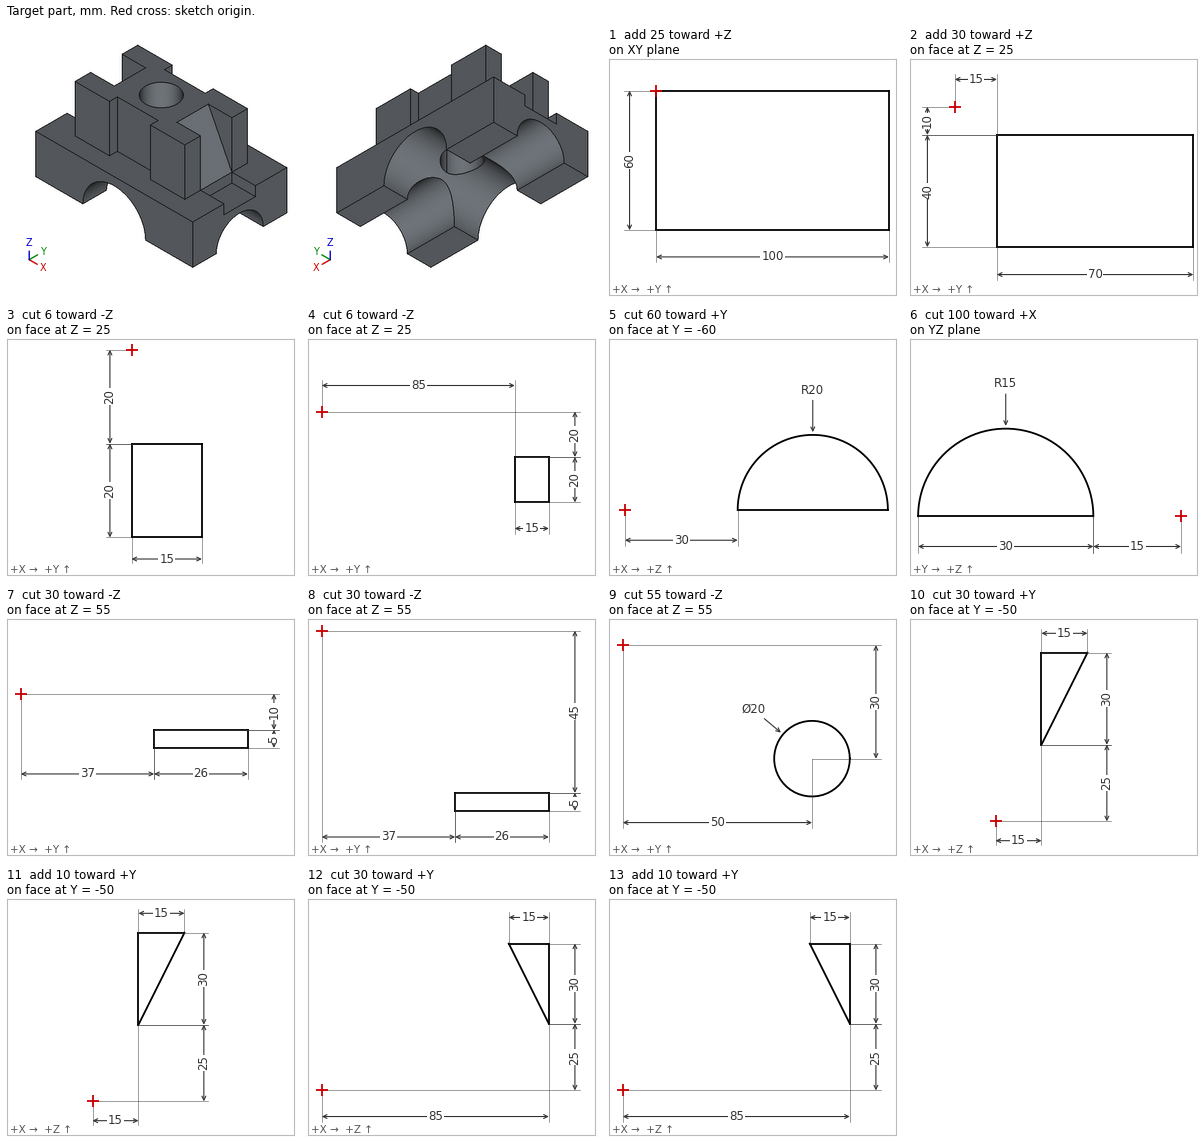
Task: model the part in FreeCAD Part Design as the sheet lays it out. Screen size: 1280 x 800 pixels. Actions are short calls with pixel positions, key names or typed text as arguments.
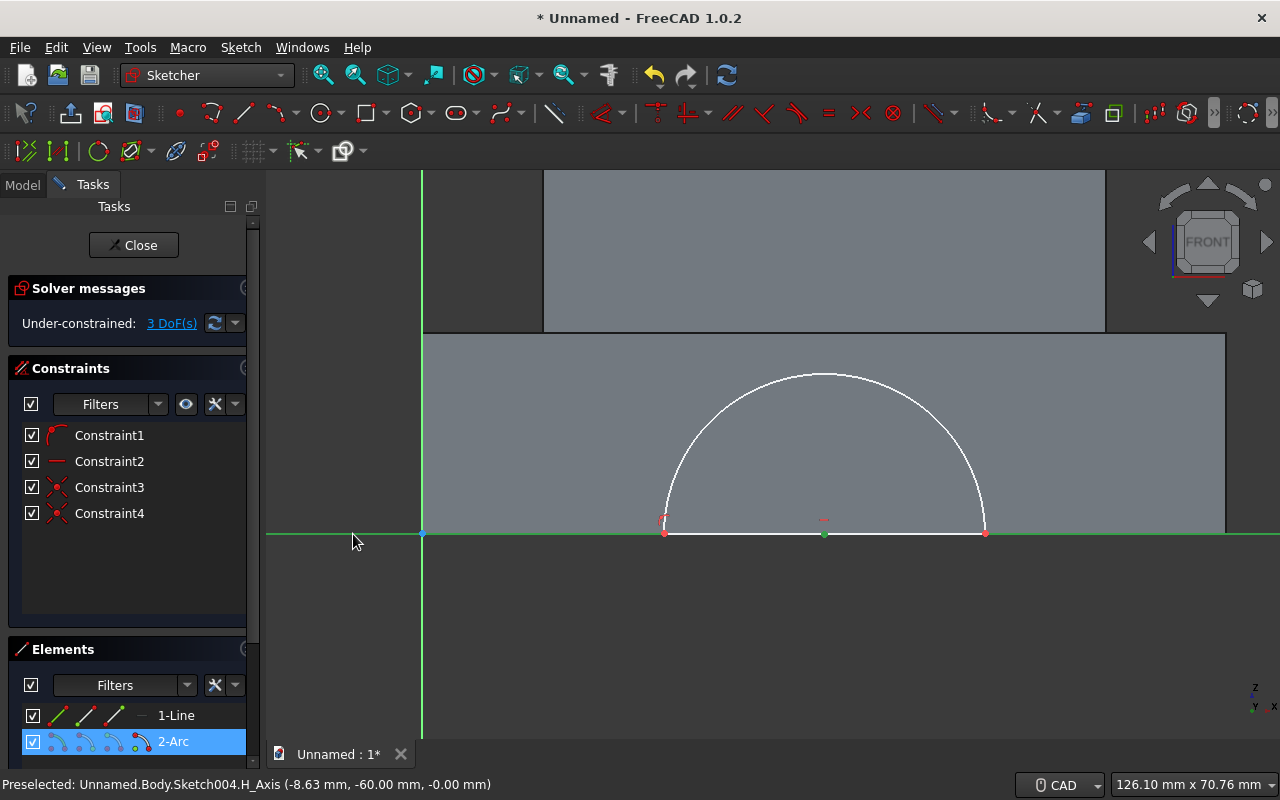
key(c)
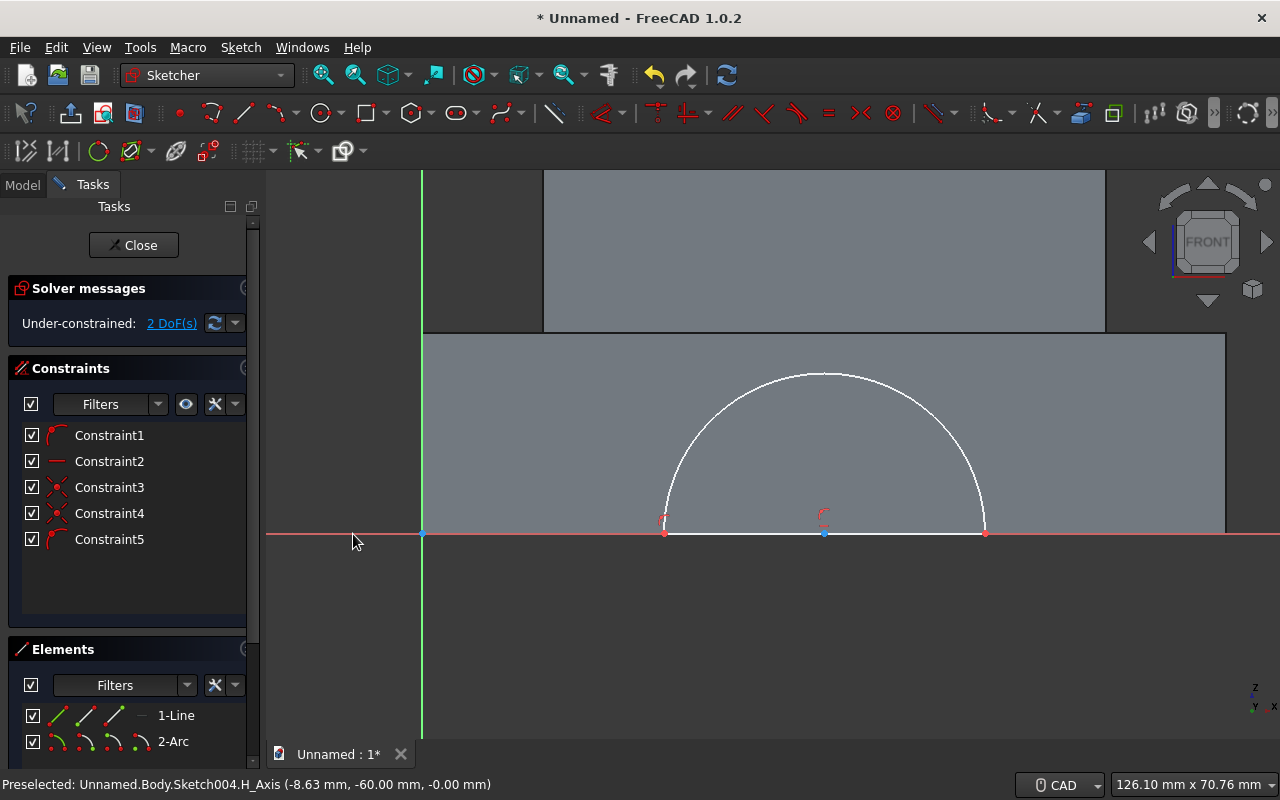
key(d)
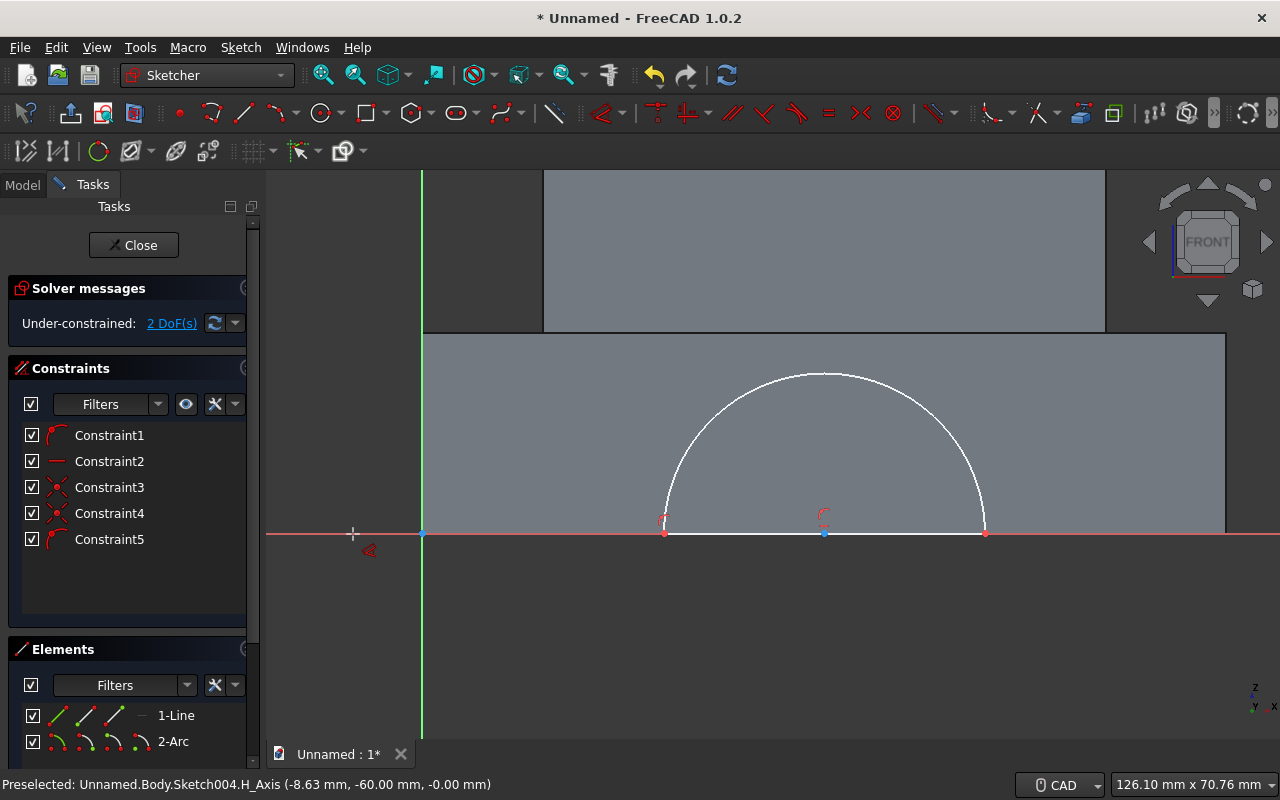
click(919, 404)
click(938, 378)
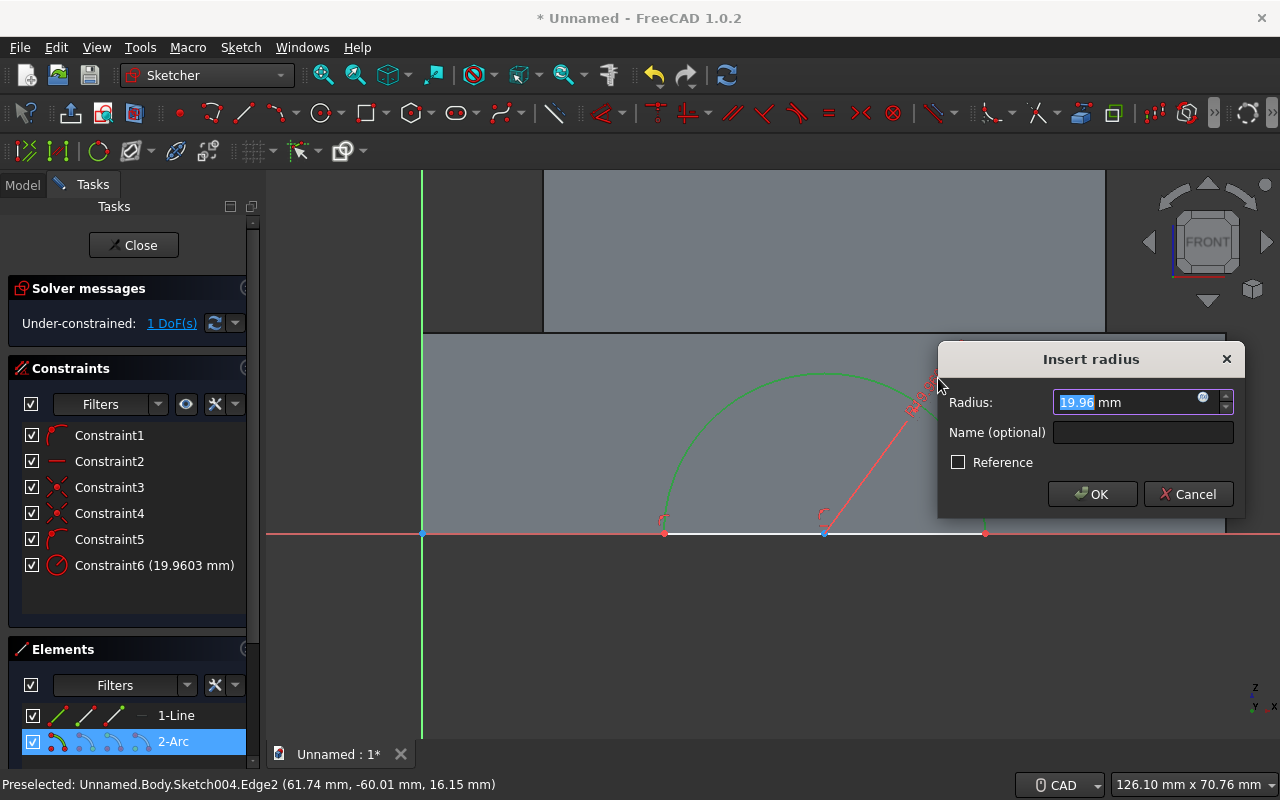
text(20)
key(Return)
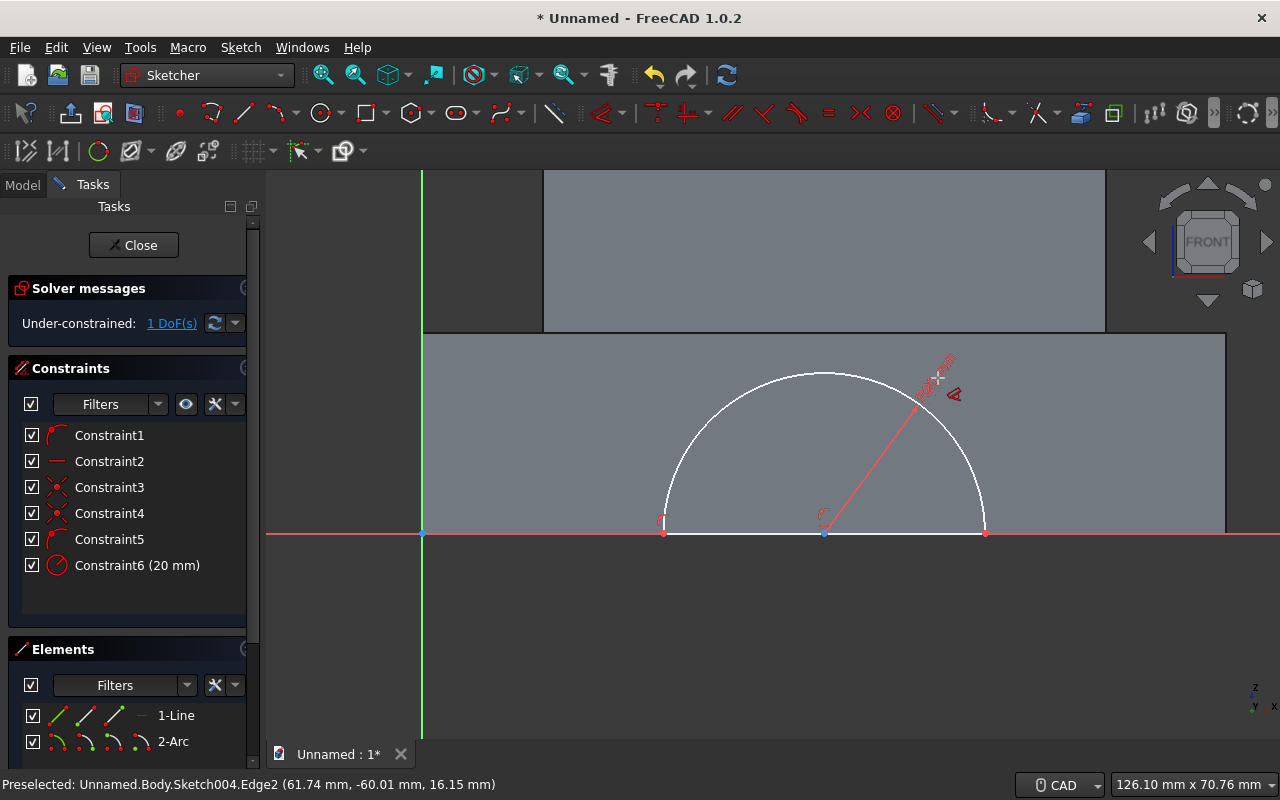
click(663, 534)
click(543, 568)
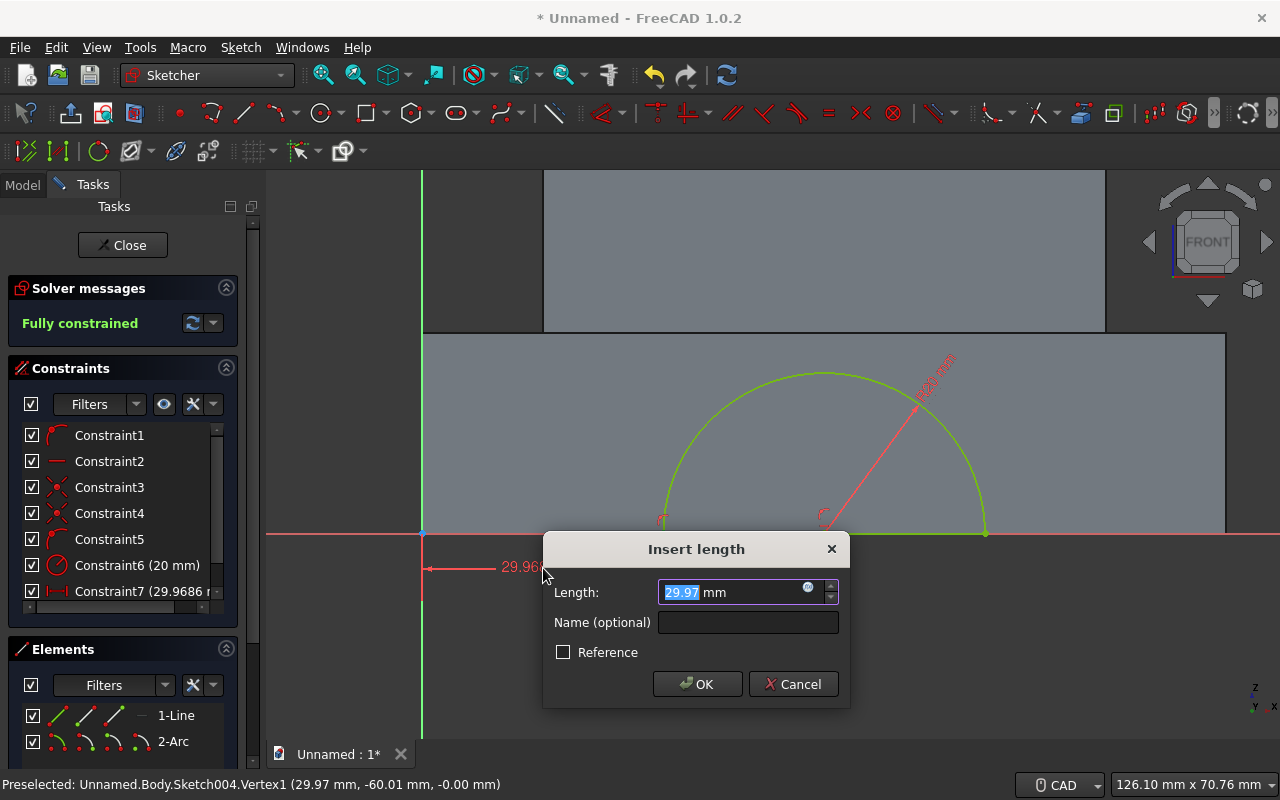
text(30)
key(Return)
key(Escape)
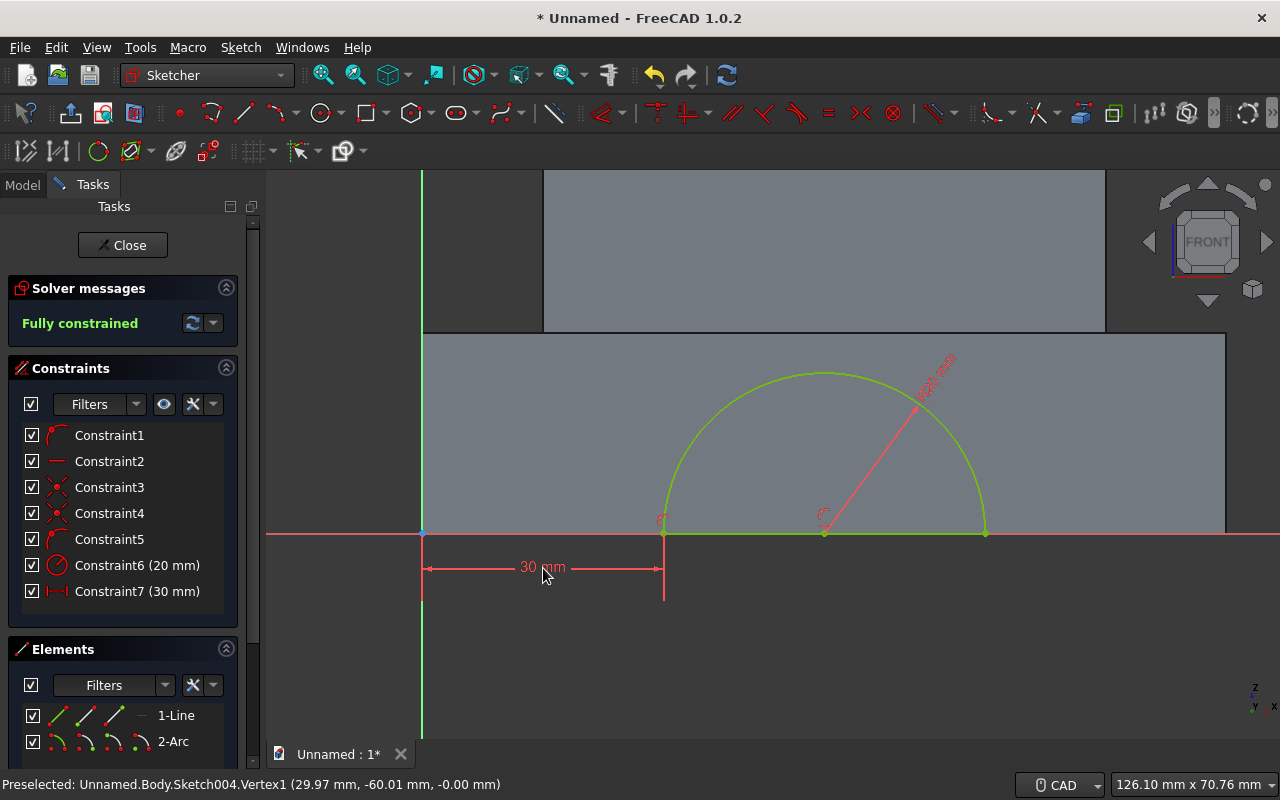
click(123, 245)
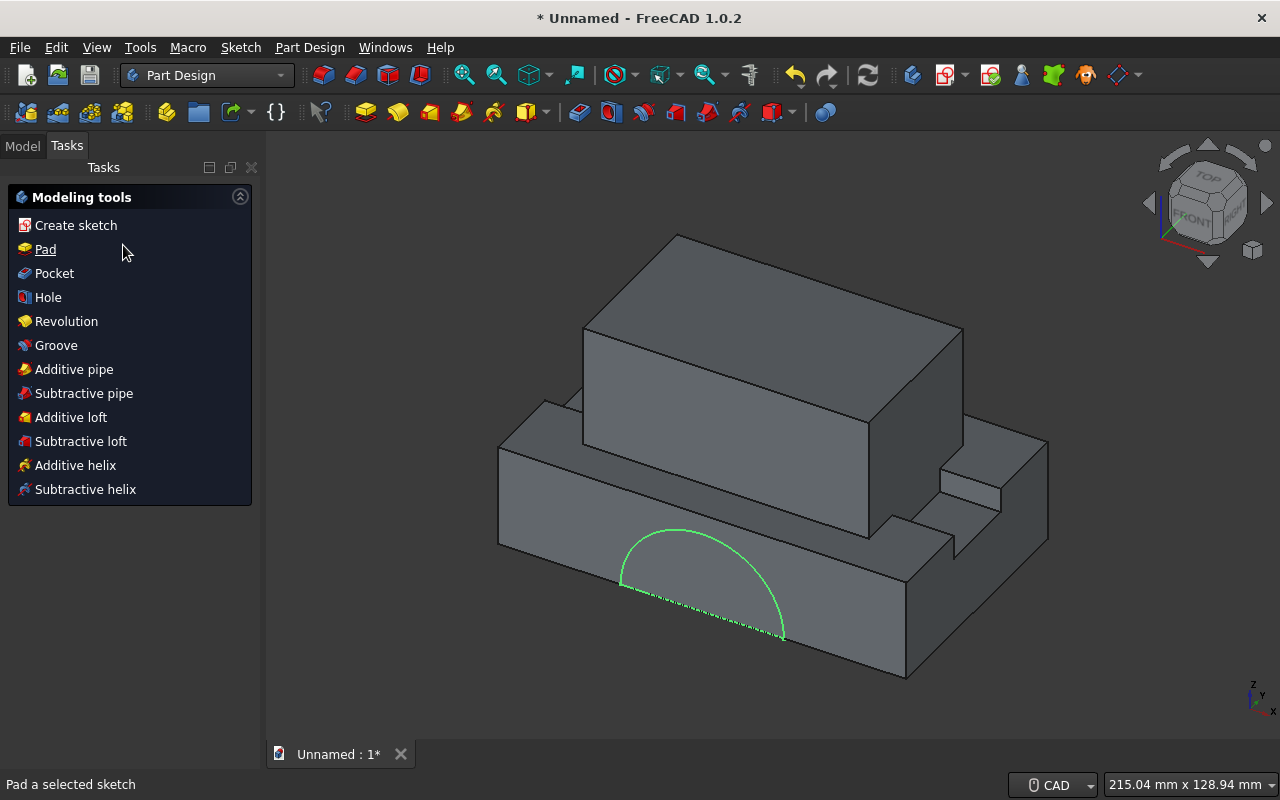
click(580, 112)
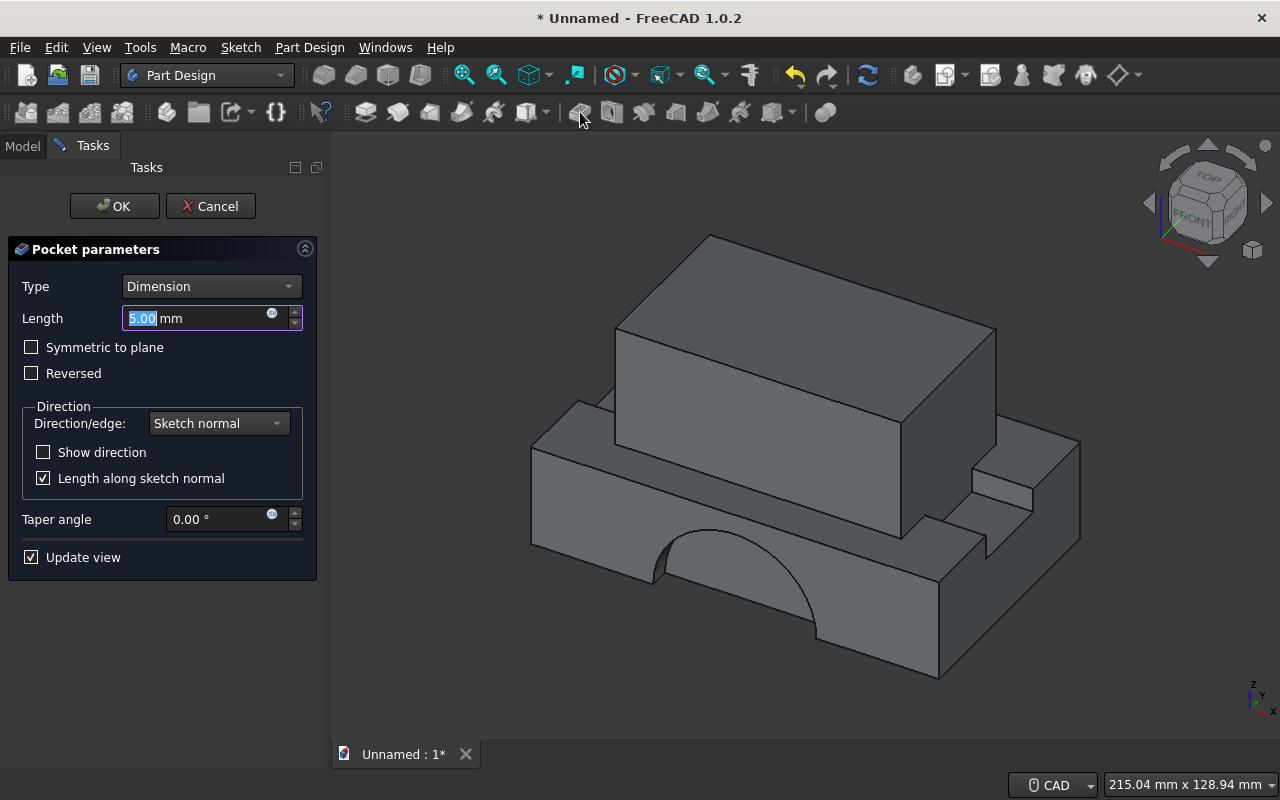
text(60)
key(Tab)